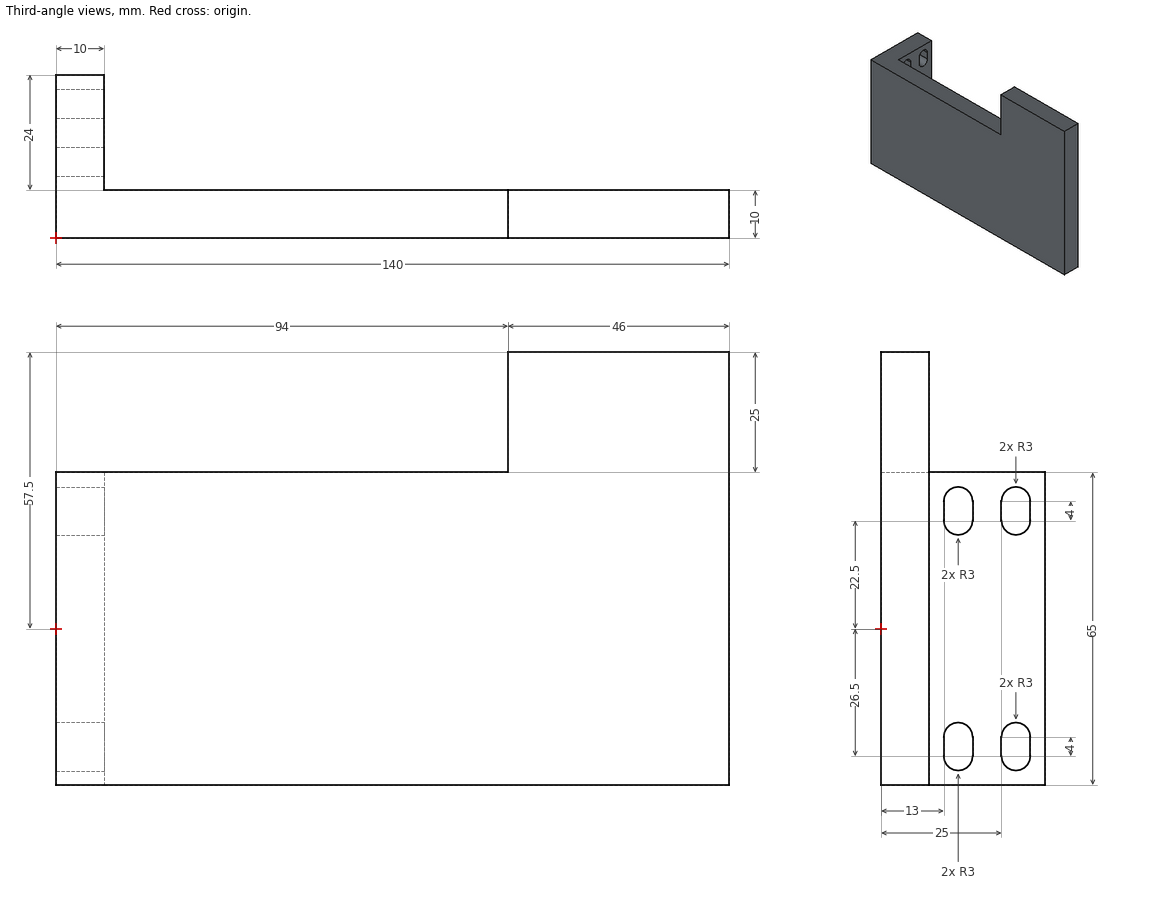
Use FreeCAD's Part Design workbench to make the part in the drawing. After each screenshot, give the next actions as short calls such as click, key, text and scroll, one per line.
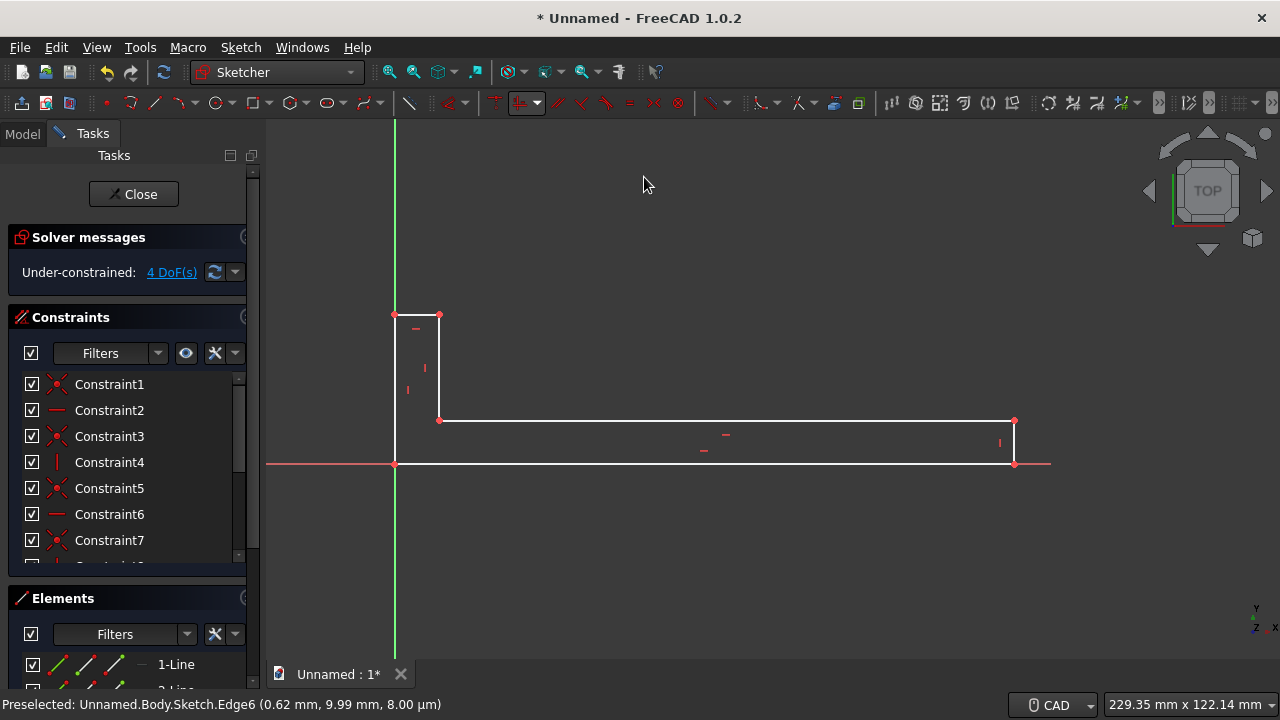
click(448, 104)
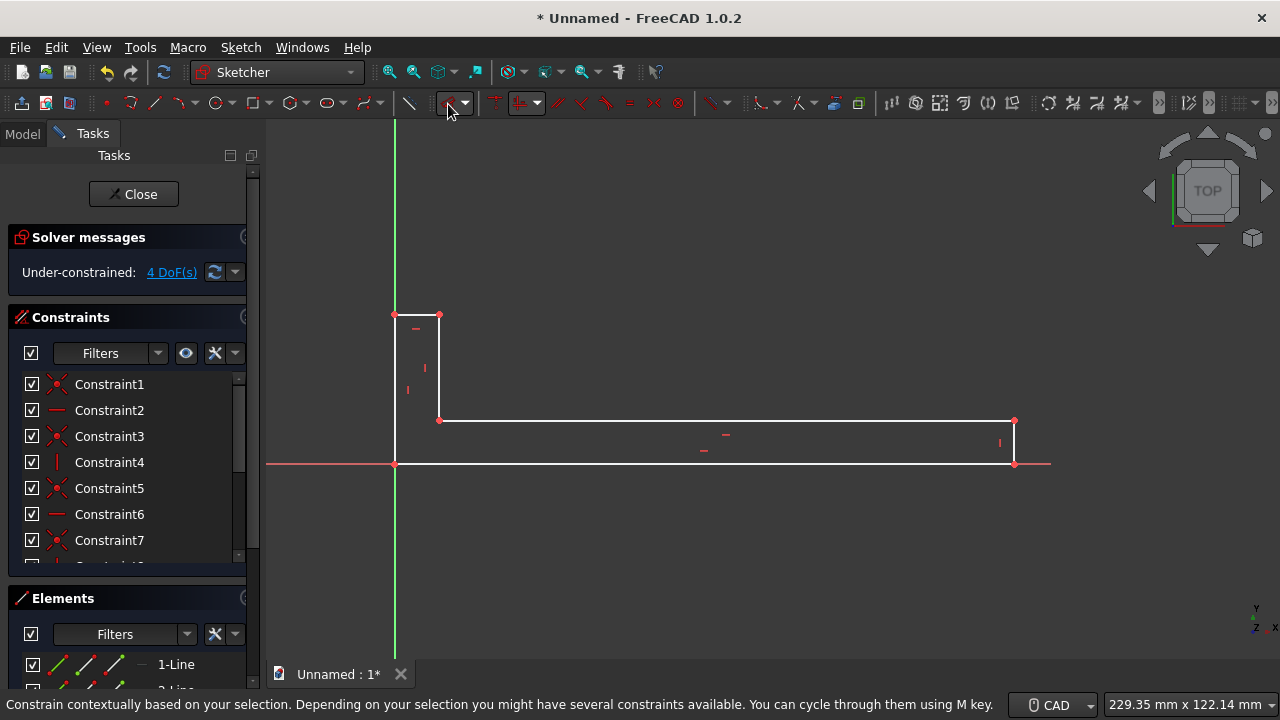
click(1014, 451)
click(1048, 443)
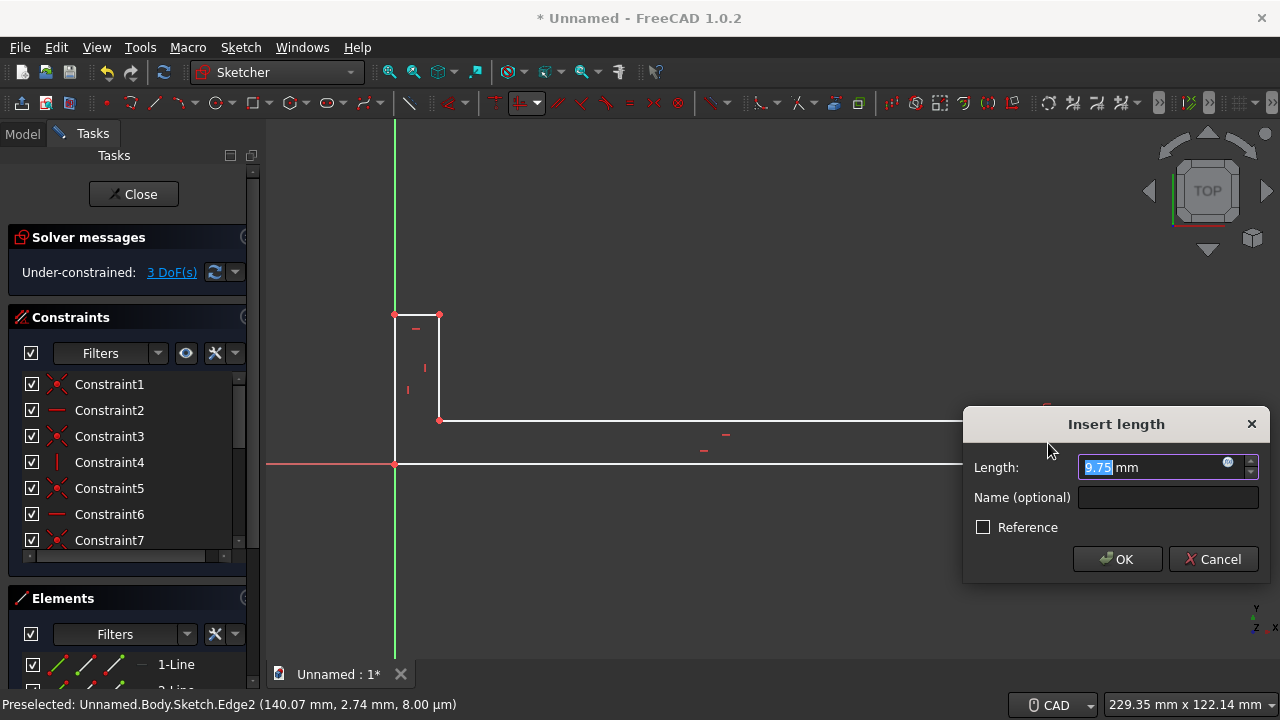
text(10)
key(Return)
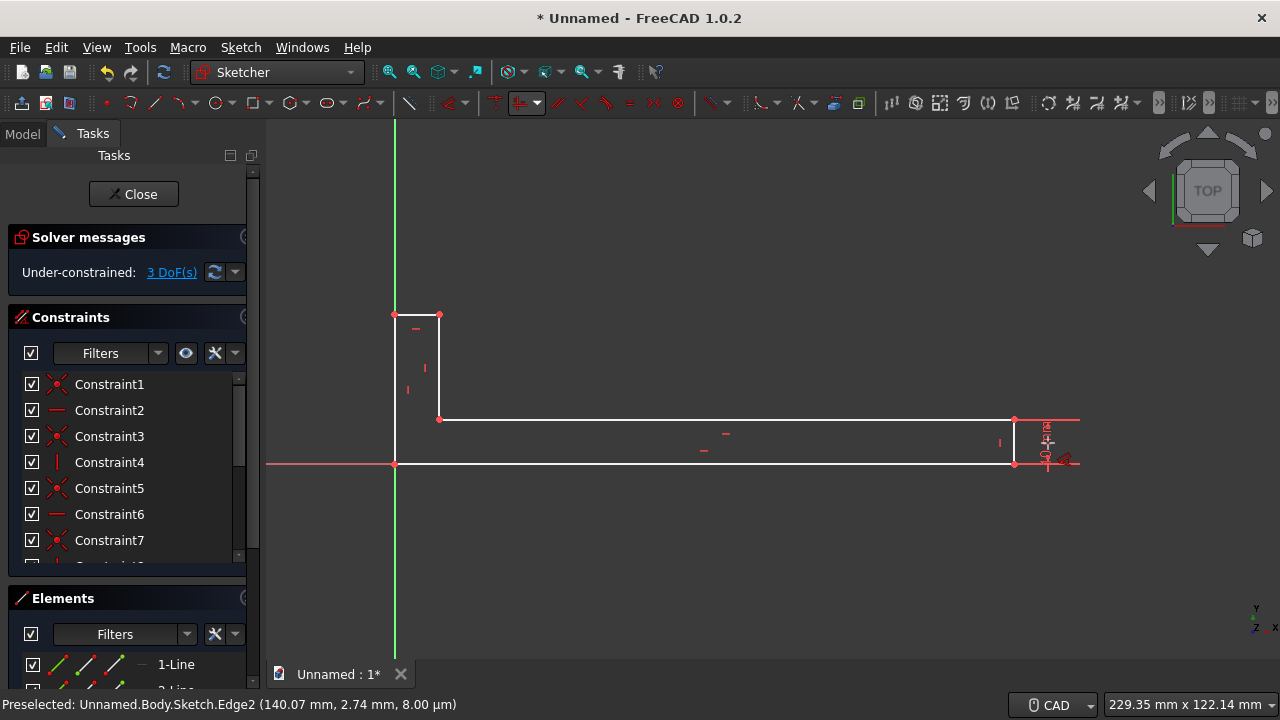
click(439, 388)
click(473, 367)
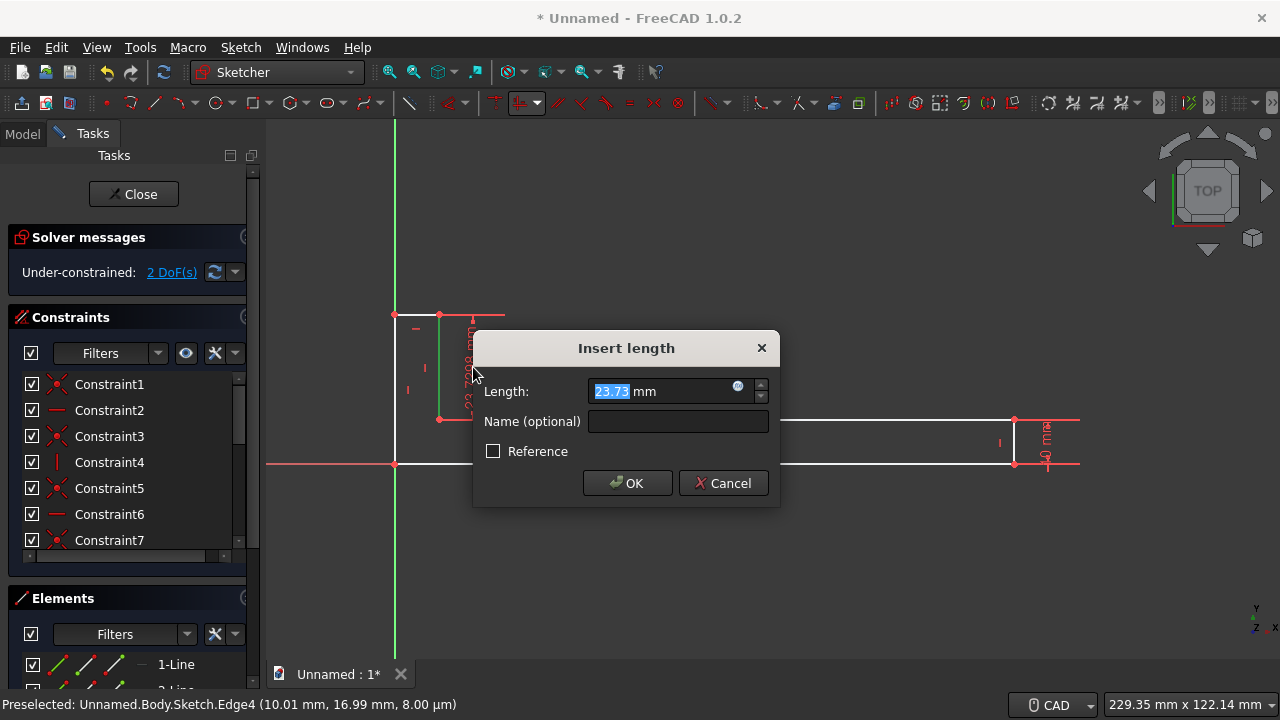
text(24)
key(Return)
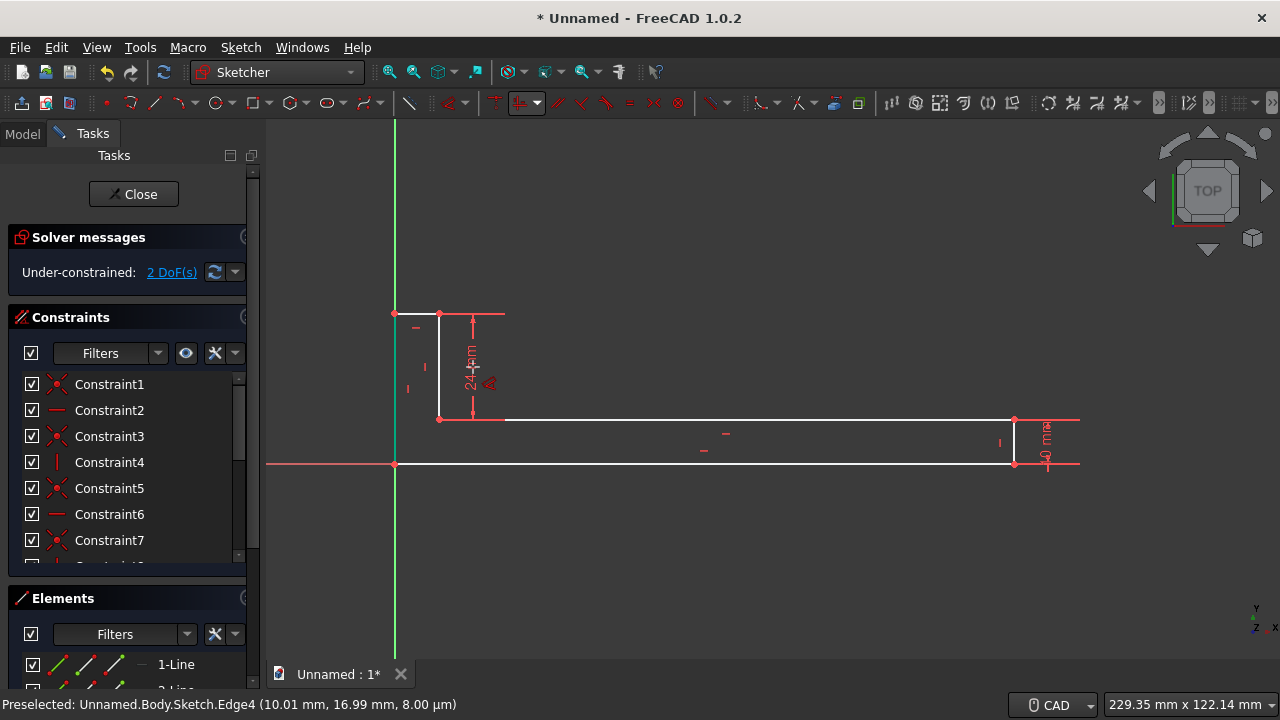
click(426, 314)
click(417, 280)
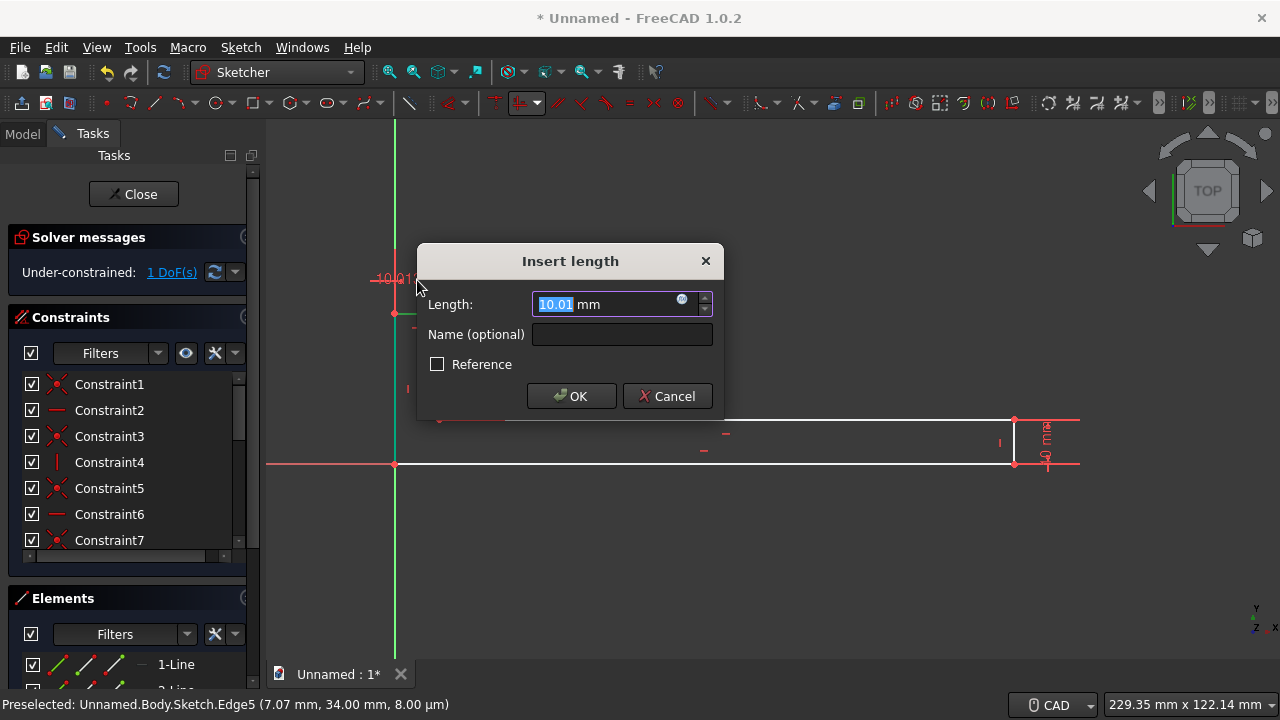
text(10)
key(Return)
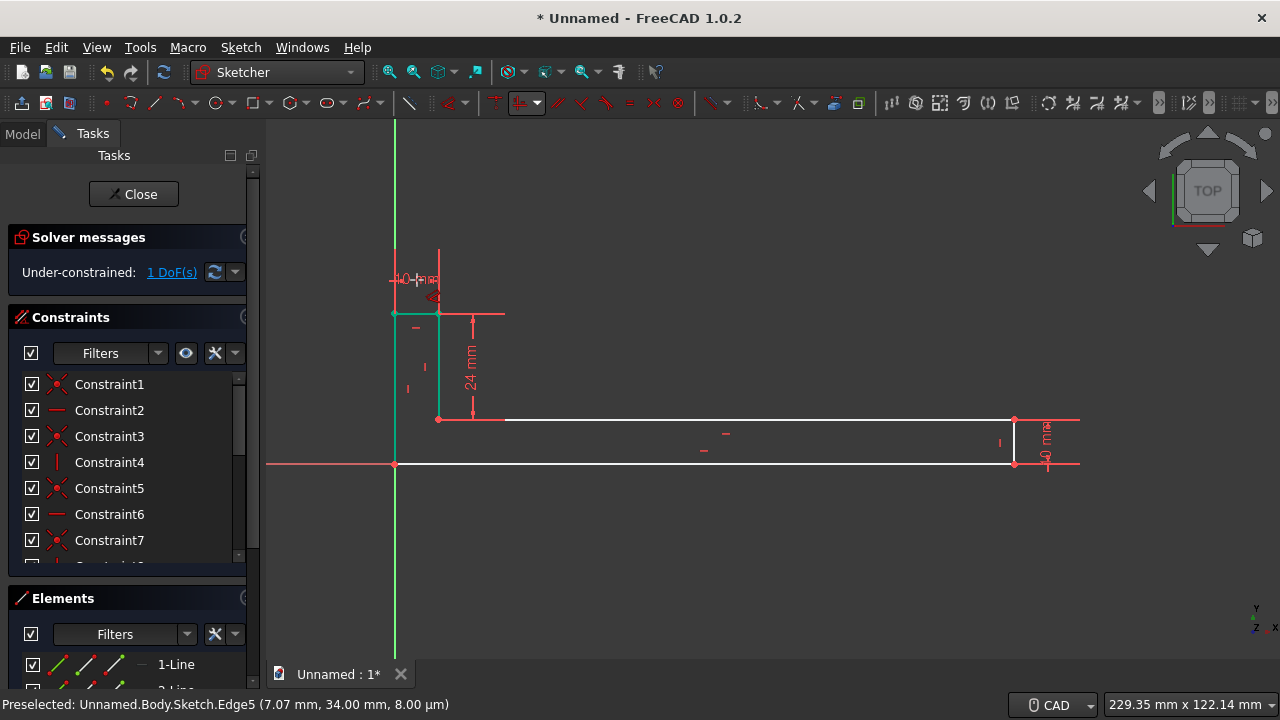
click(581, 464)
click(704, 498)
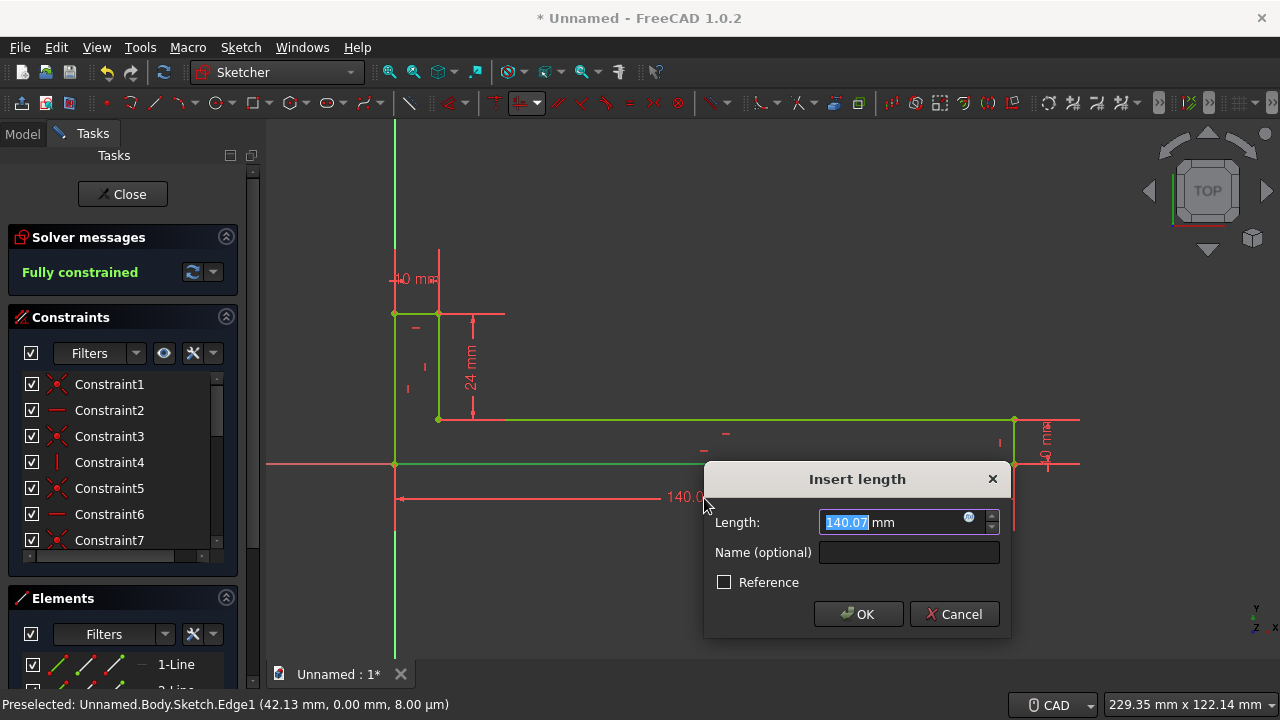
text(140)
key(Return)
key(Escape)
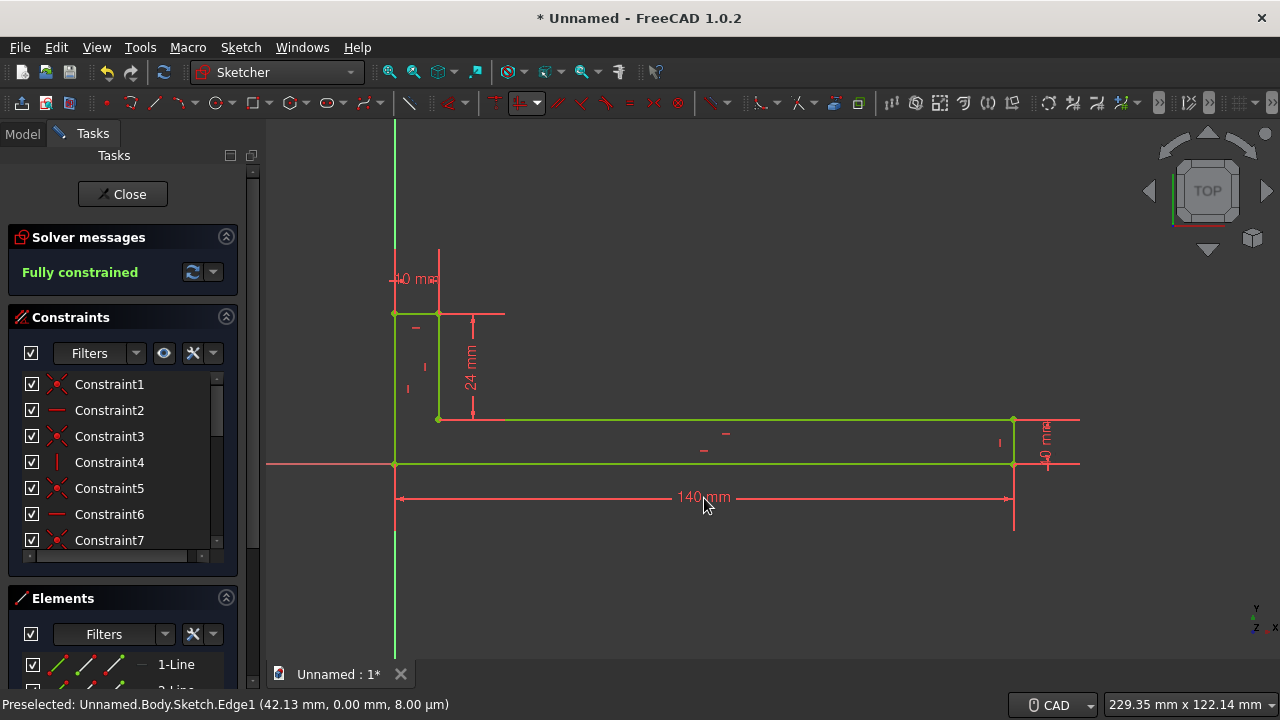
click(123, 194)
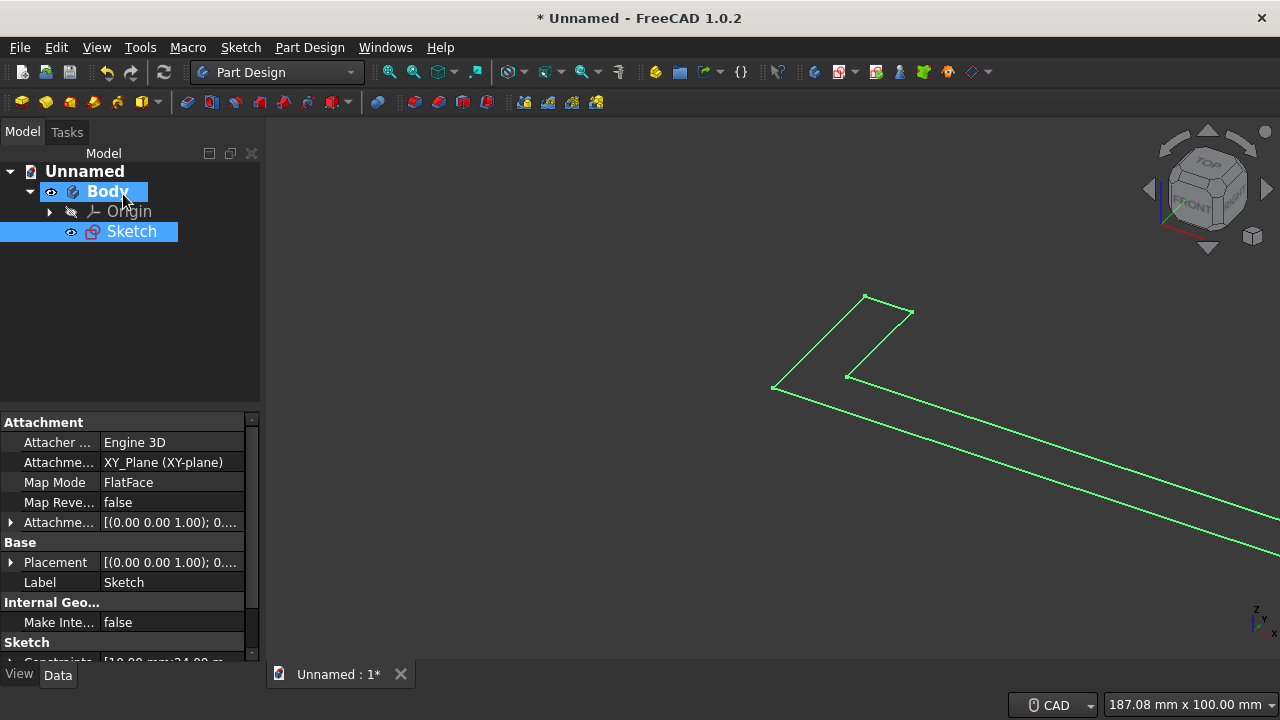
click(22, 102)